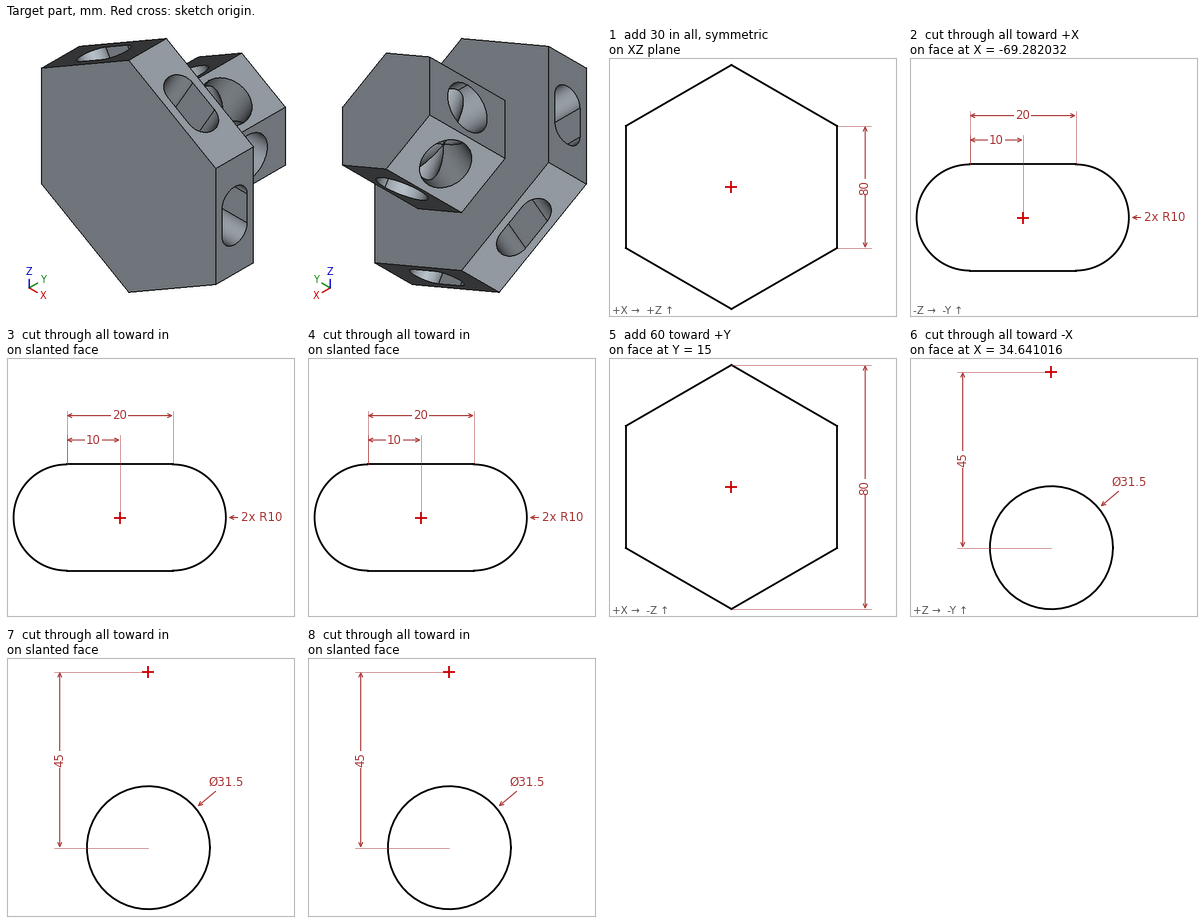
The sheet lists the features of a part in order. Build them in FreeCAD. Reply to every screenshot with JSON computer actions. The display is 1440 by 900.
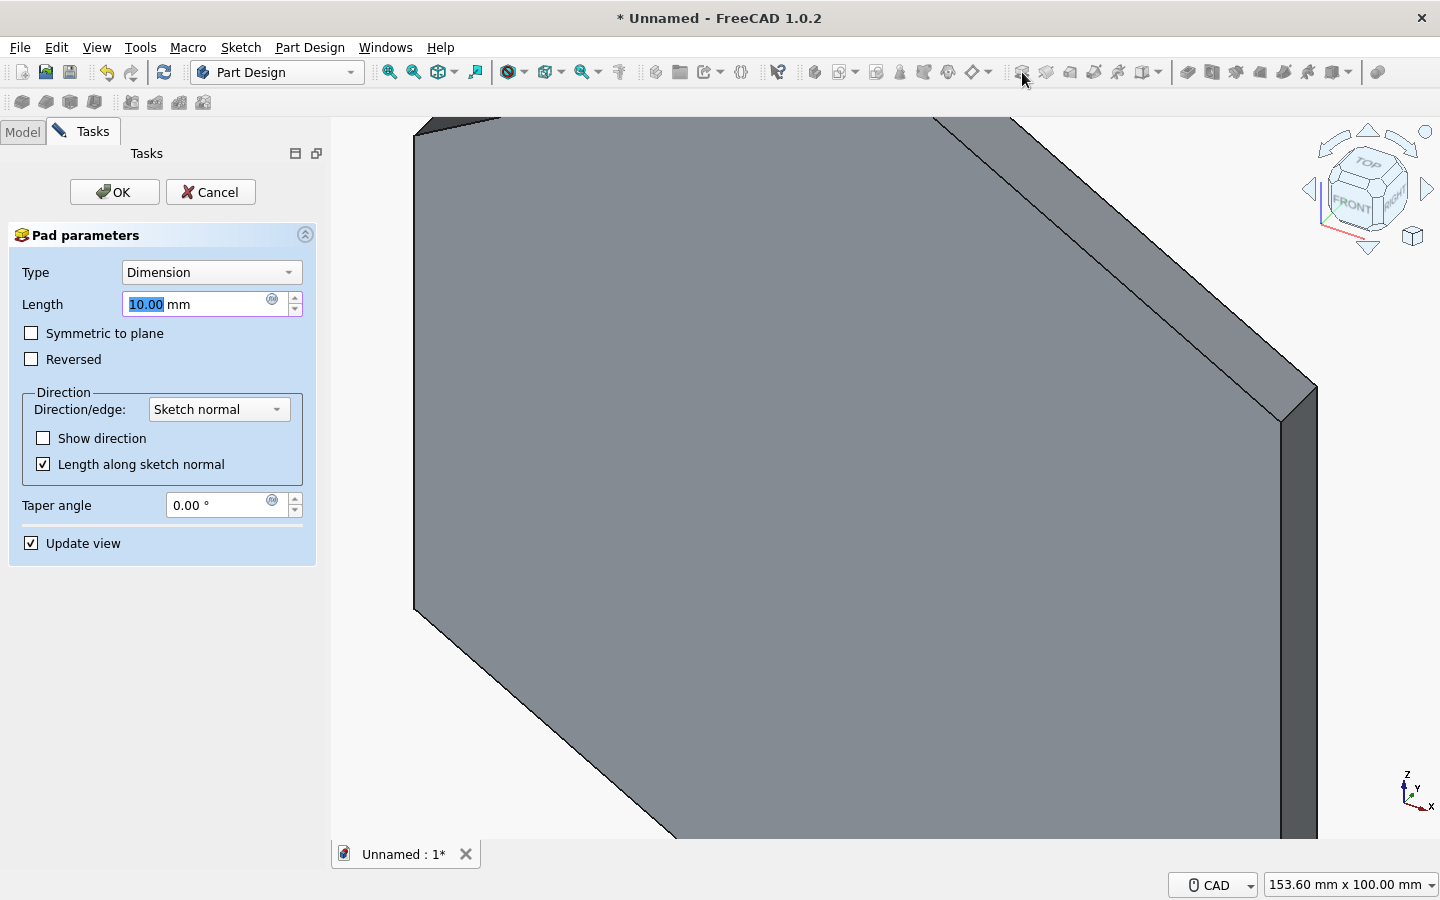
{"action": "type", "text": "30"}
{"action": "key", "text": "Tab"}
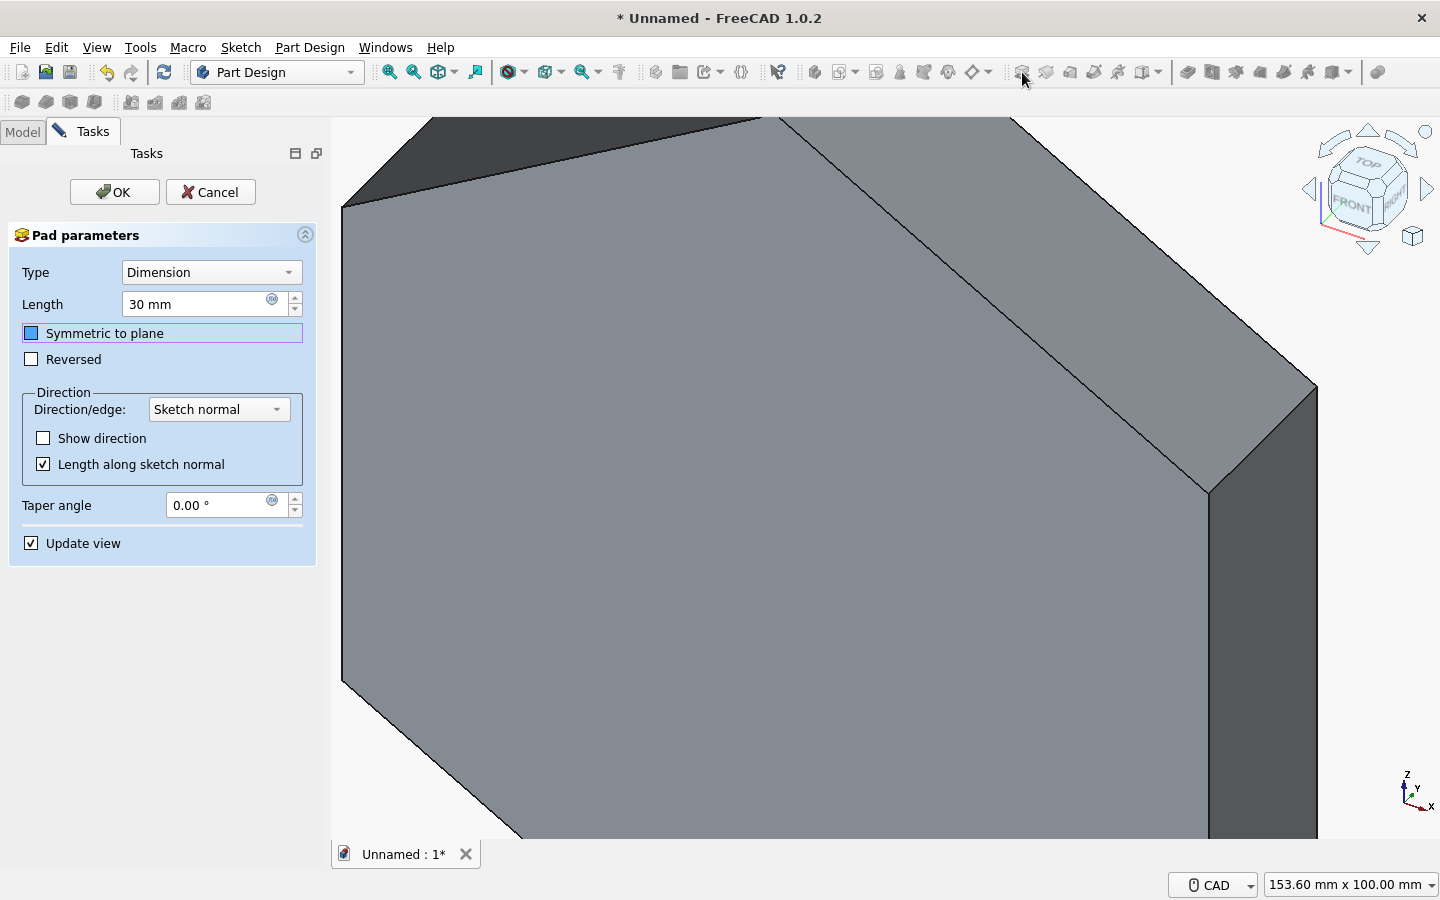
{"action": "left_click", "coordinate": [30, 333]}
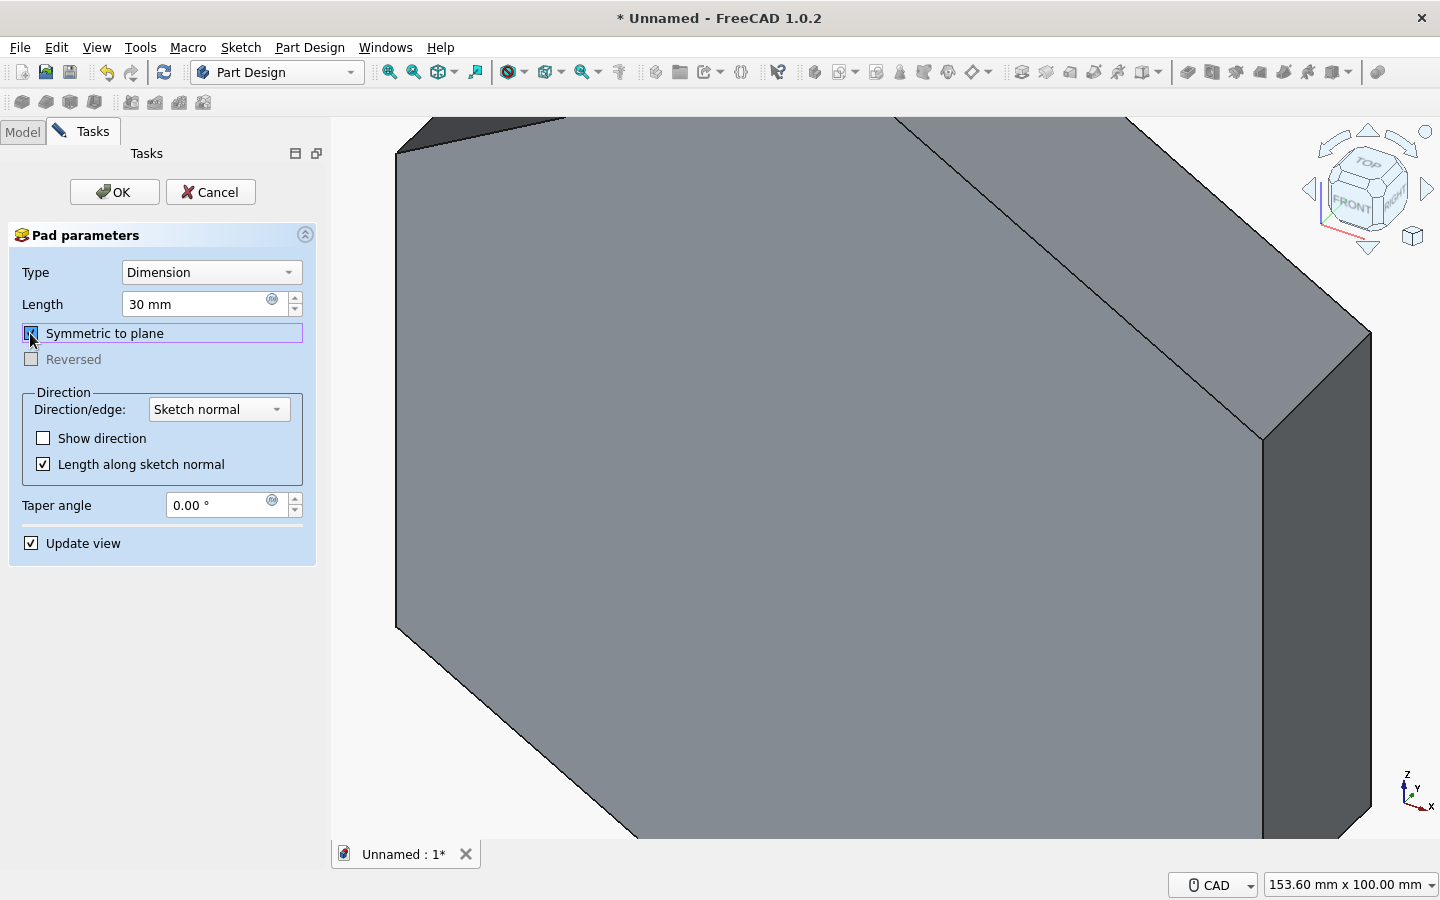
{"action": "left_click", "coordinate": [115, 192]}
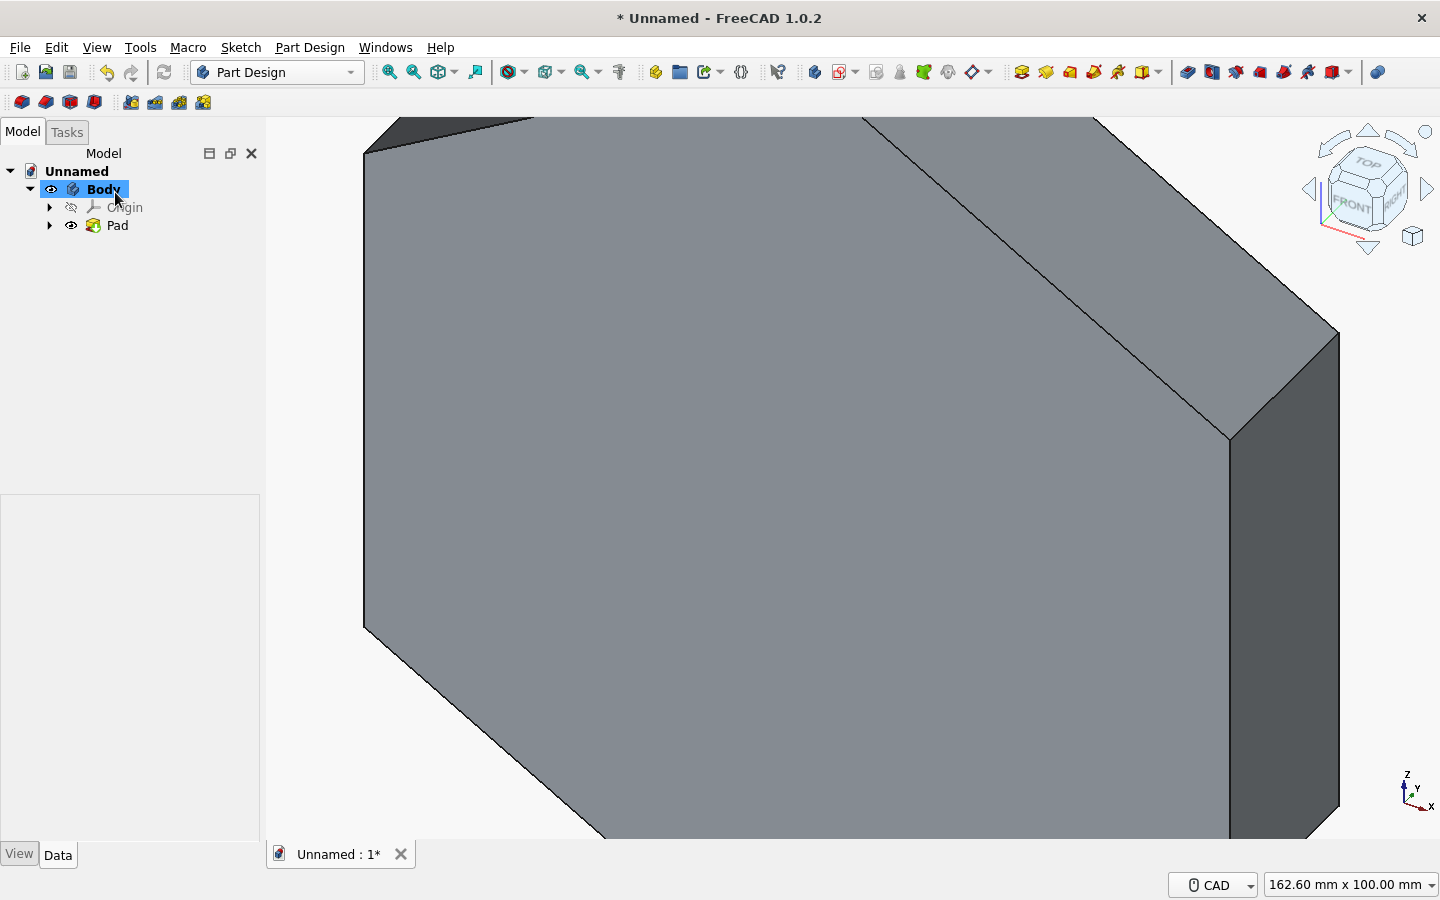
{"action": "left_click", "coordinate": [390, 72]}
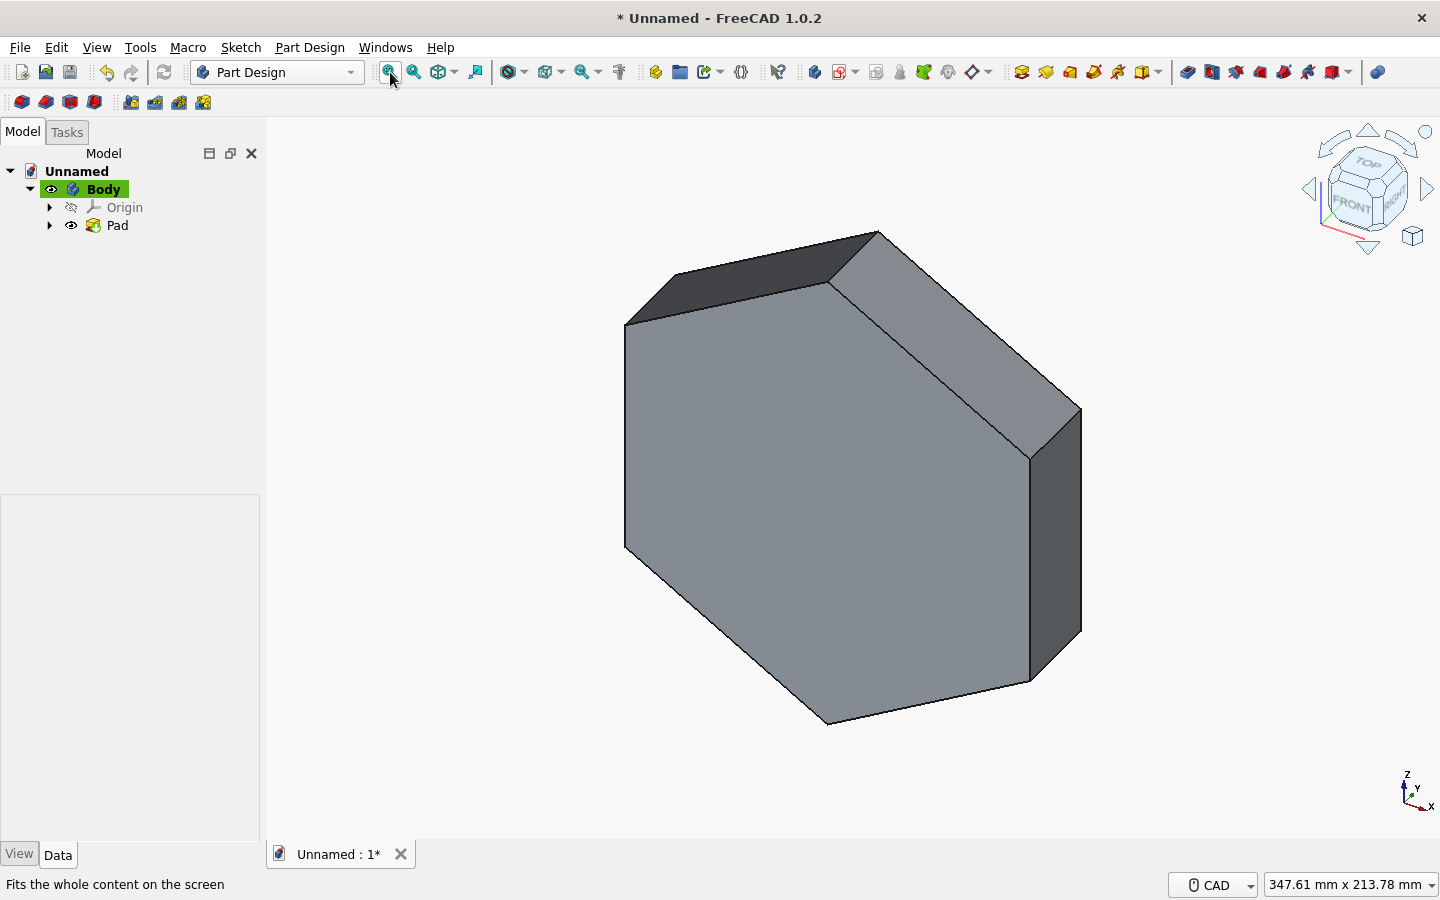
{"action": "key", "text": "6"}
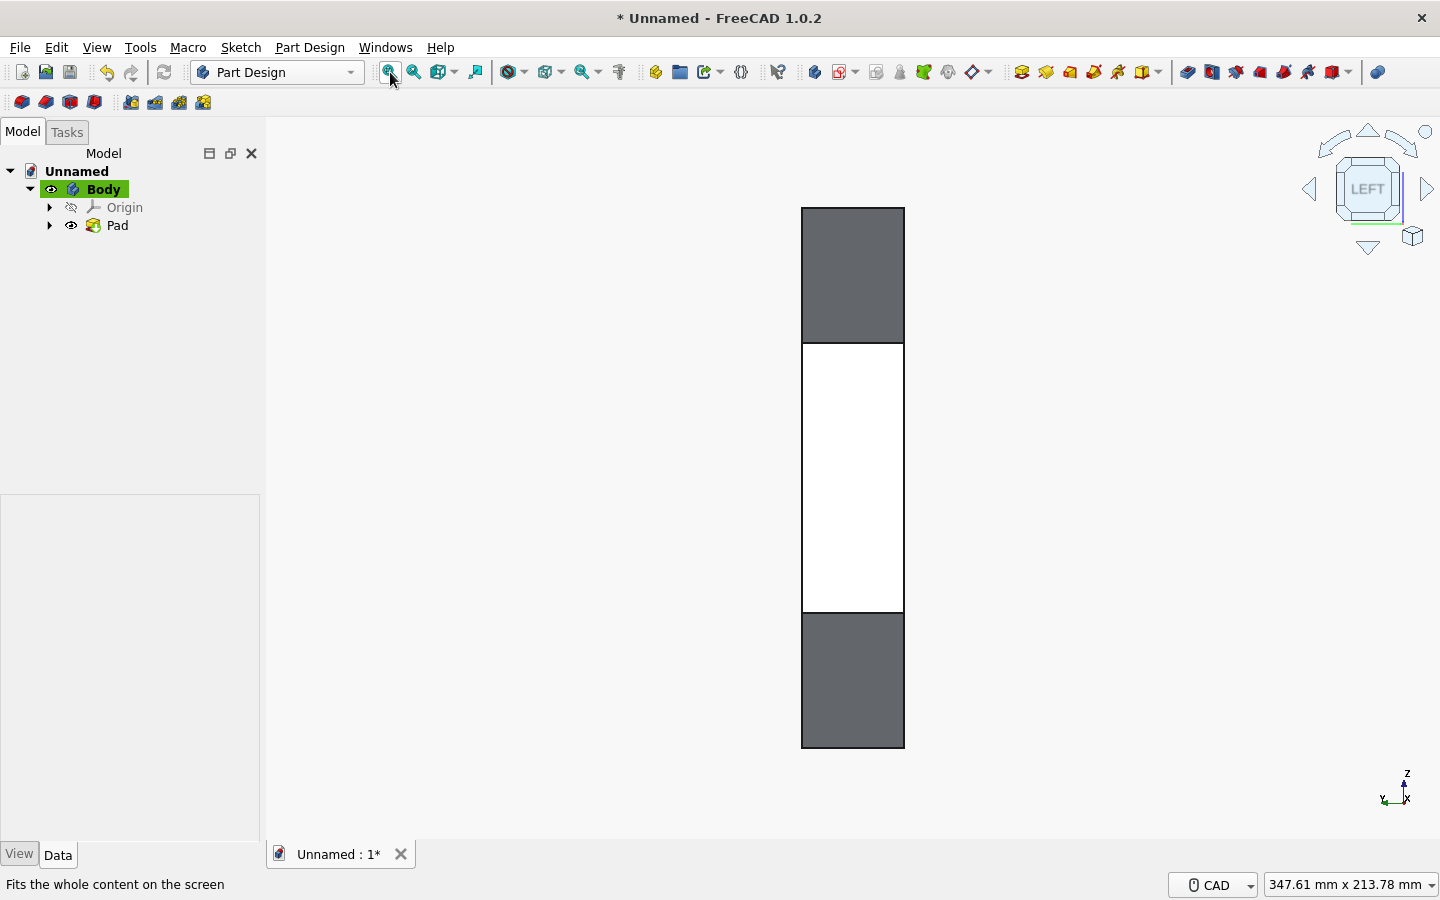
{"action": "left_click", "coordinate": [853, 477]}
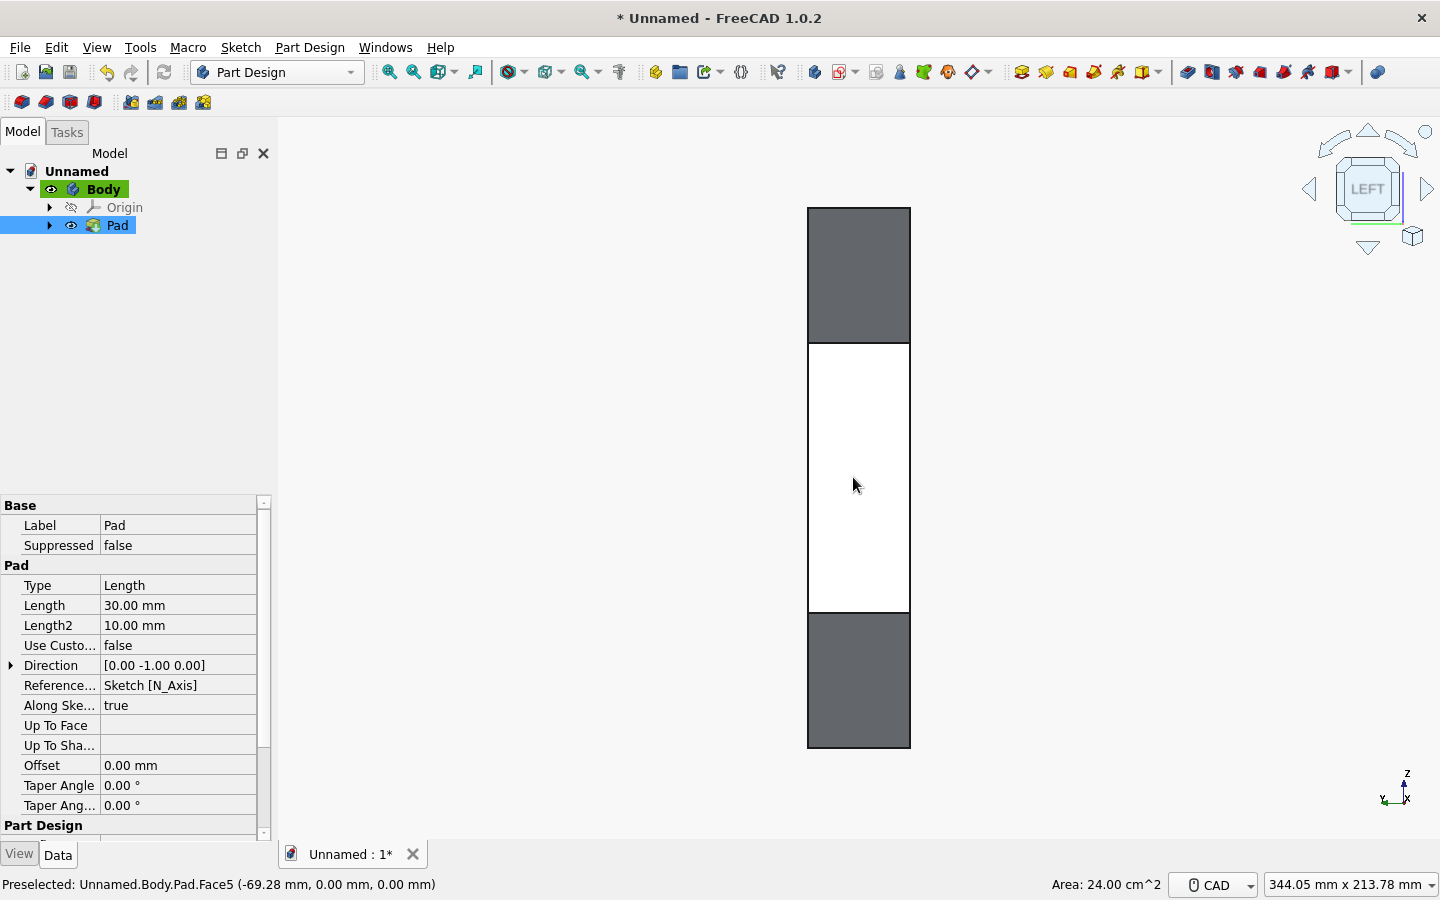
{"action": "left_click", "coordinate": [840, 72]}